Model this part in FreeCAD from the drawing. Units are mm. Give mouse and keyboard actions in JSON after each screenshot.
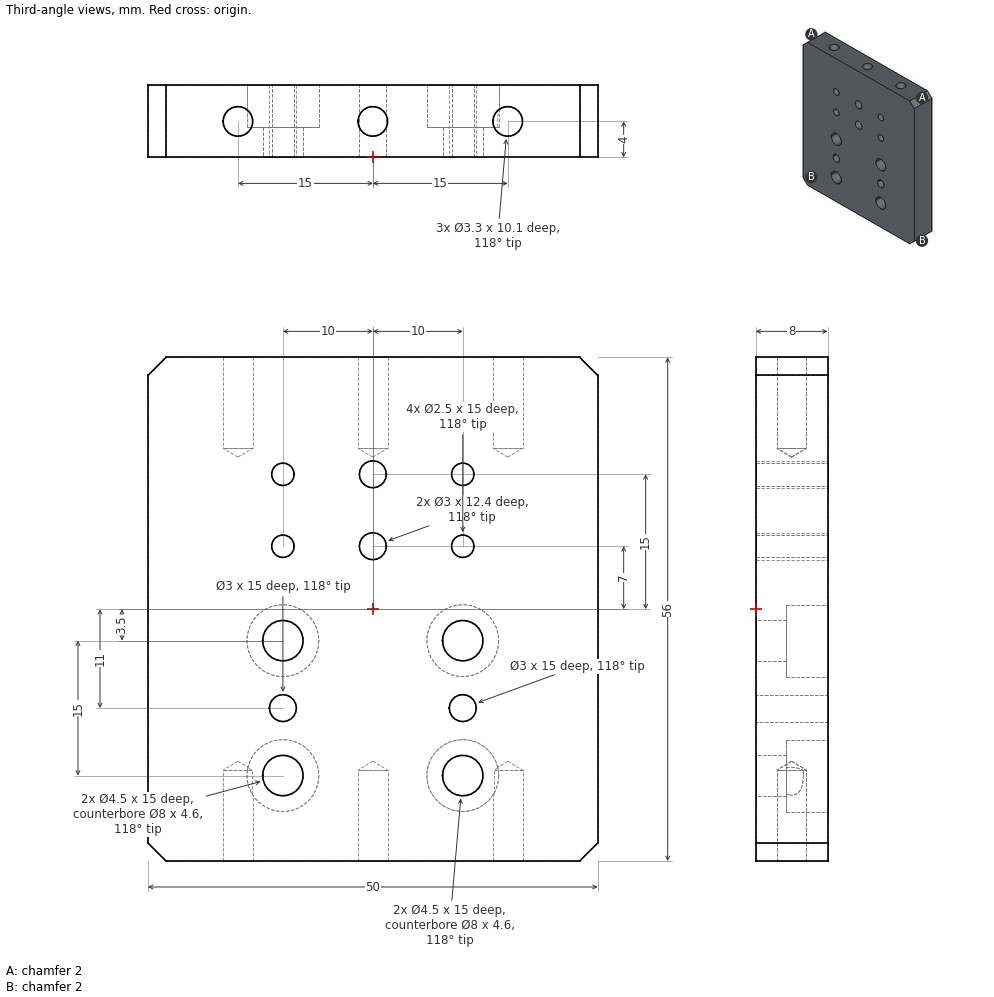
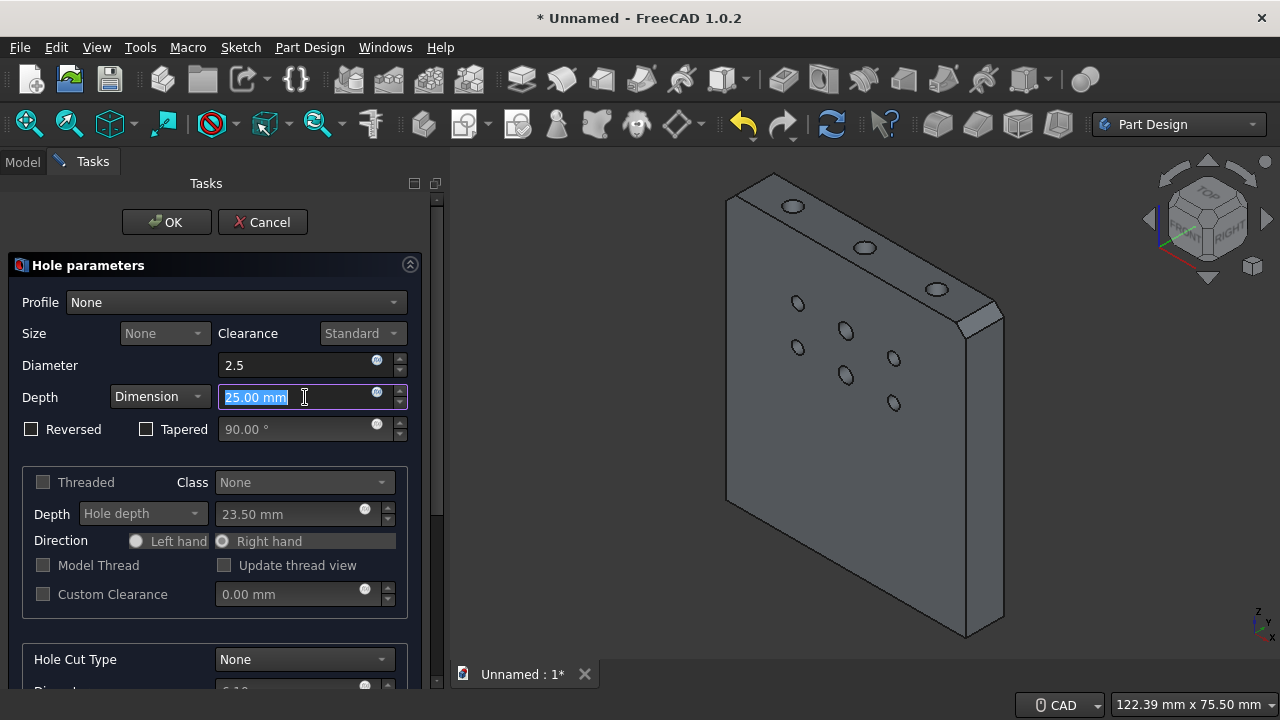
{"action": "type", "text": "15"}
{"action": "key", "text": "Tab"}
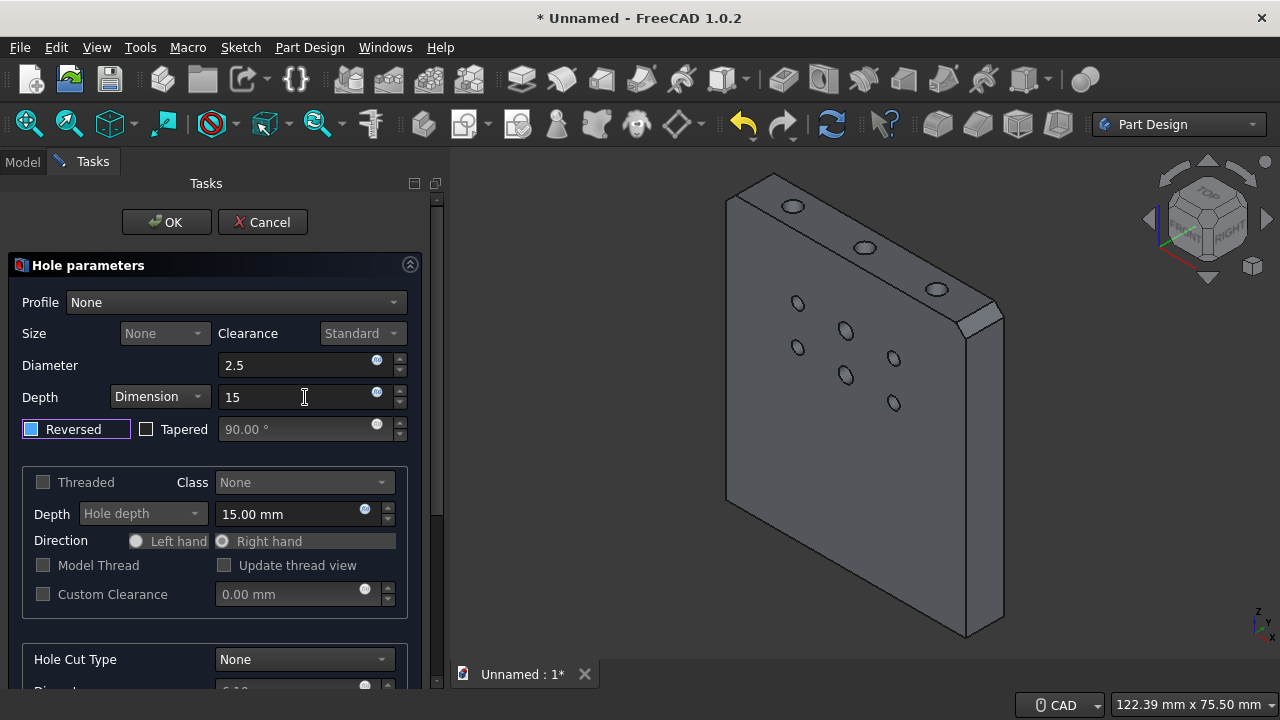
{"action": "left_click", "coordinate": [167, 222]}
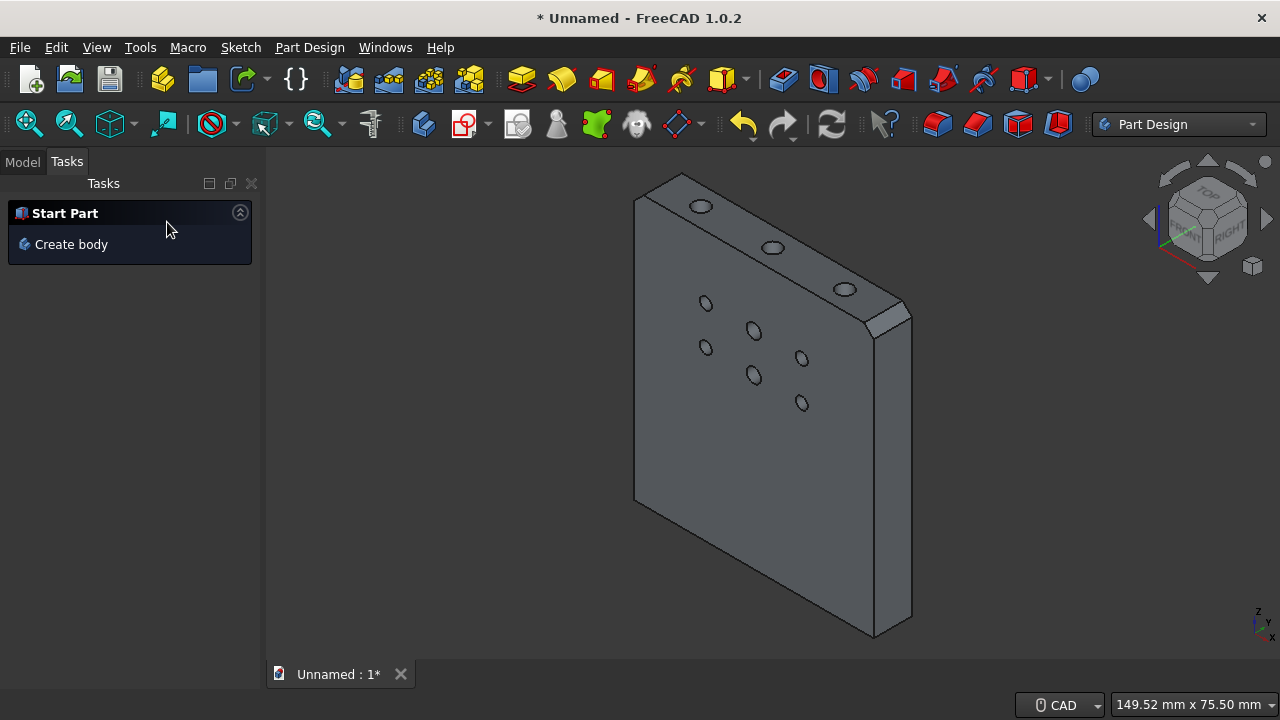
{"action": "key", "text": "4"}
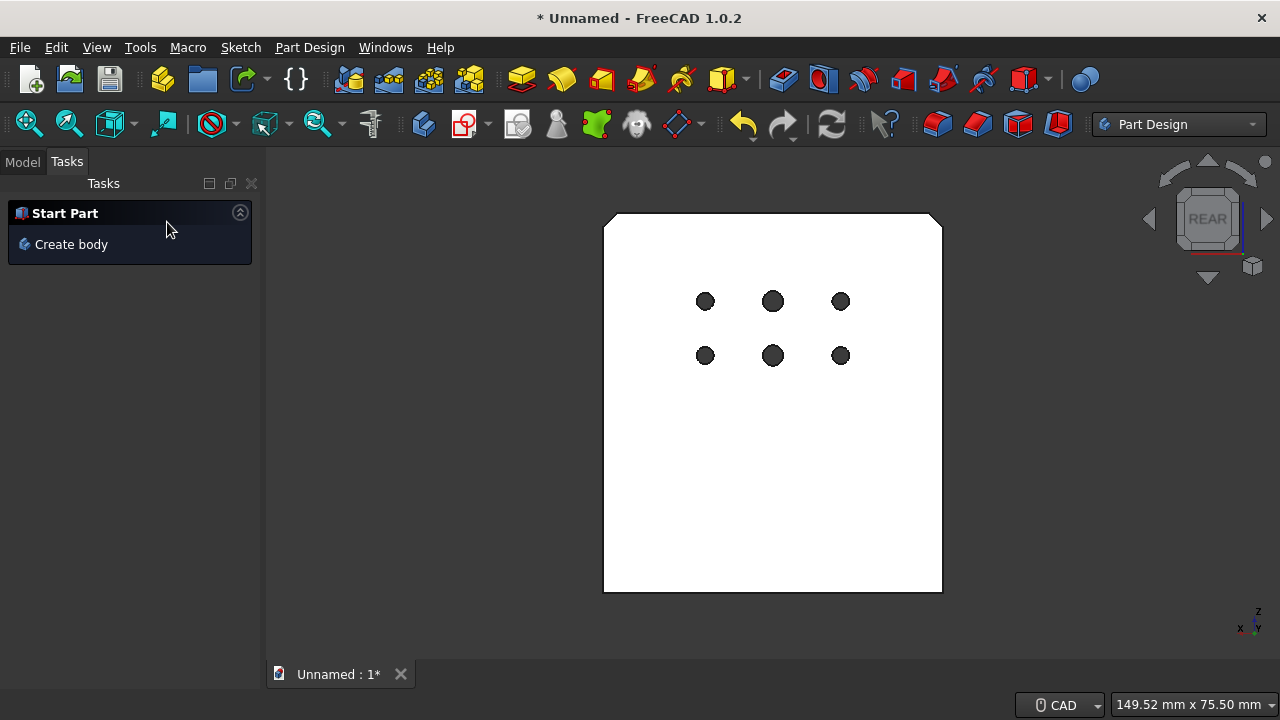
{"action": "left_click", "coordinate": [725, 456]}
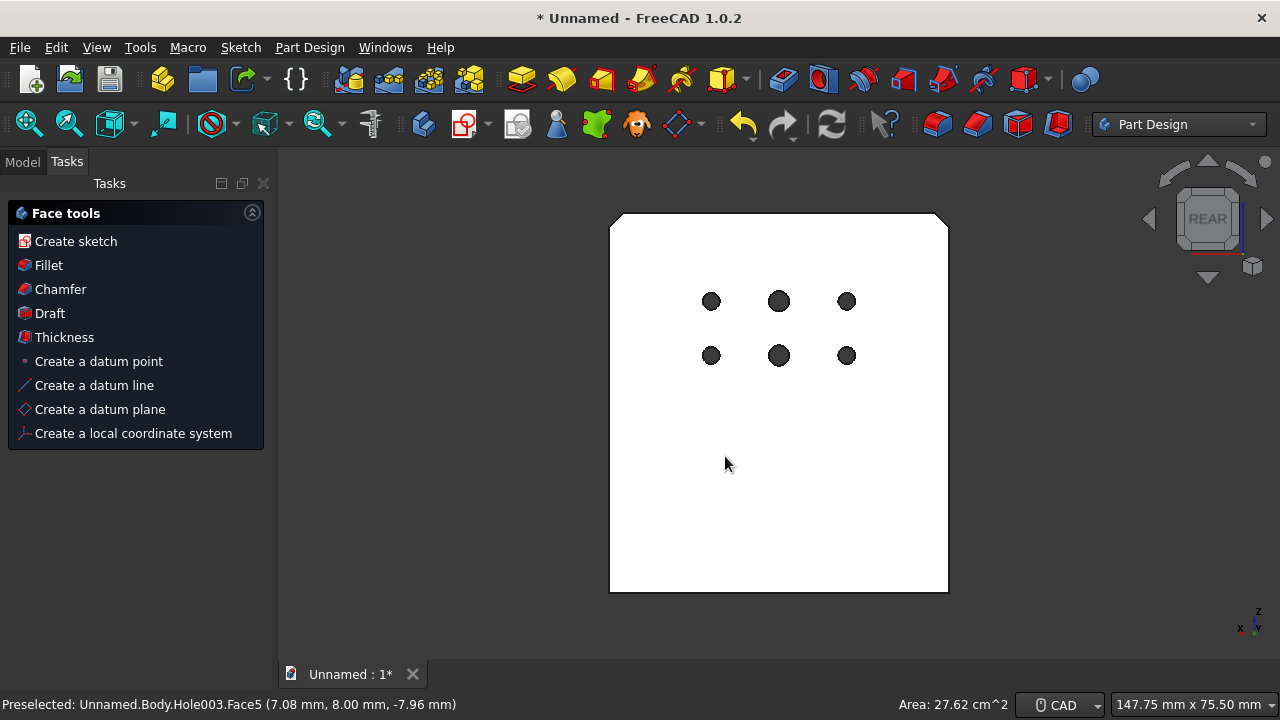
{"action": "left_click", "coordinate": [464, 124]}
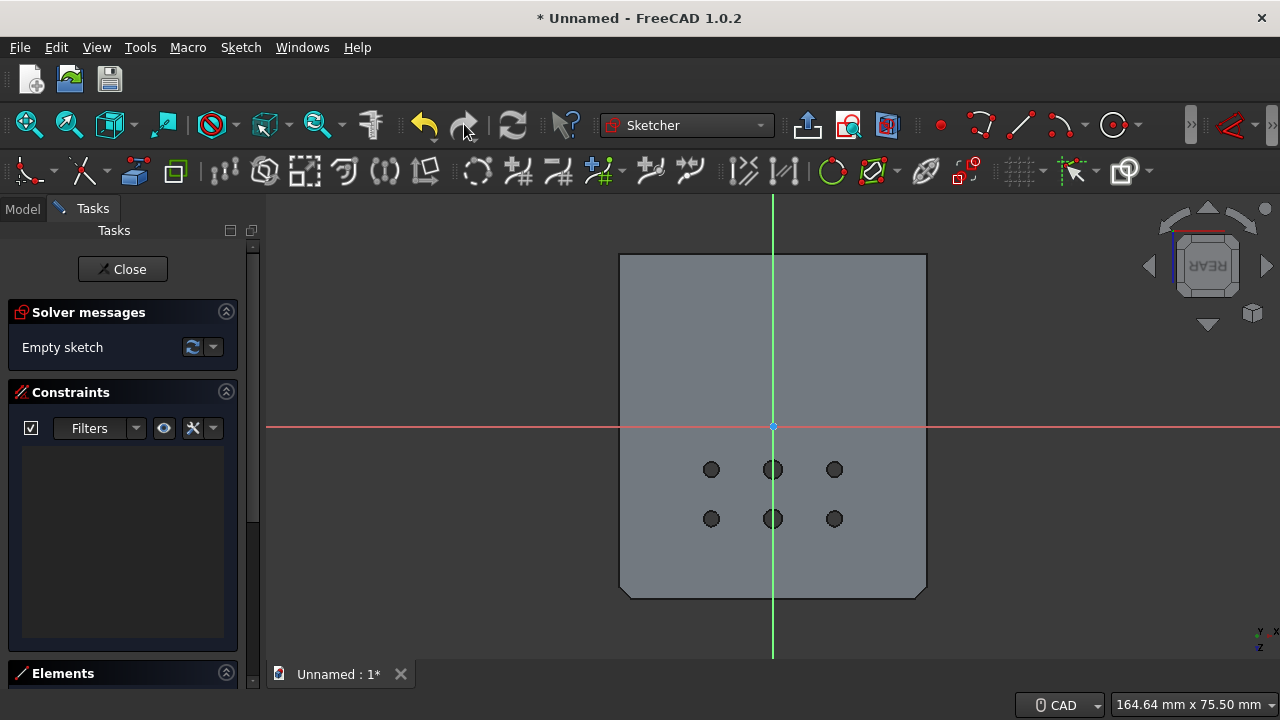
{"action": "scroll", "coordinate": [712, 354], "scroll_direction": "up", "scroll_amount": 14}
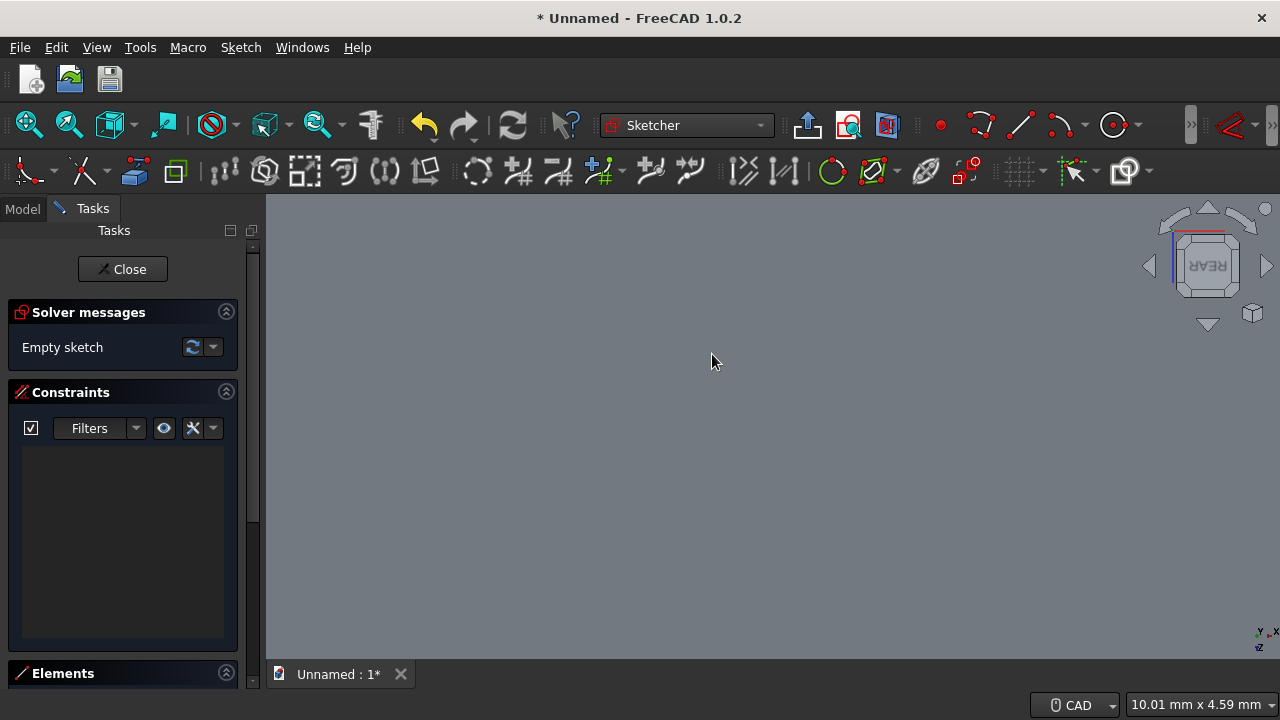
{"action": "key", "text": "g c"}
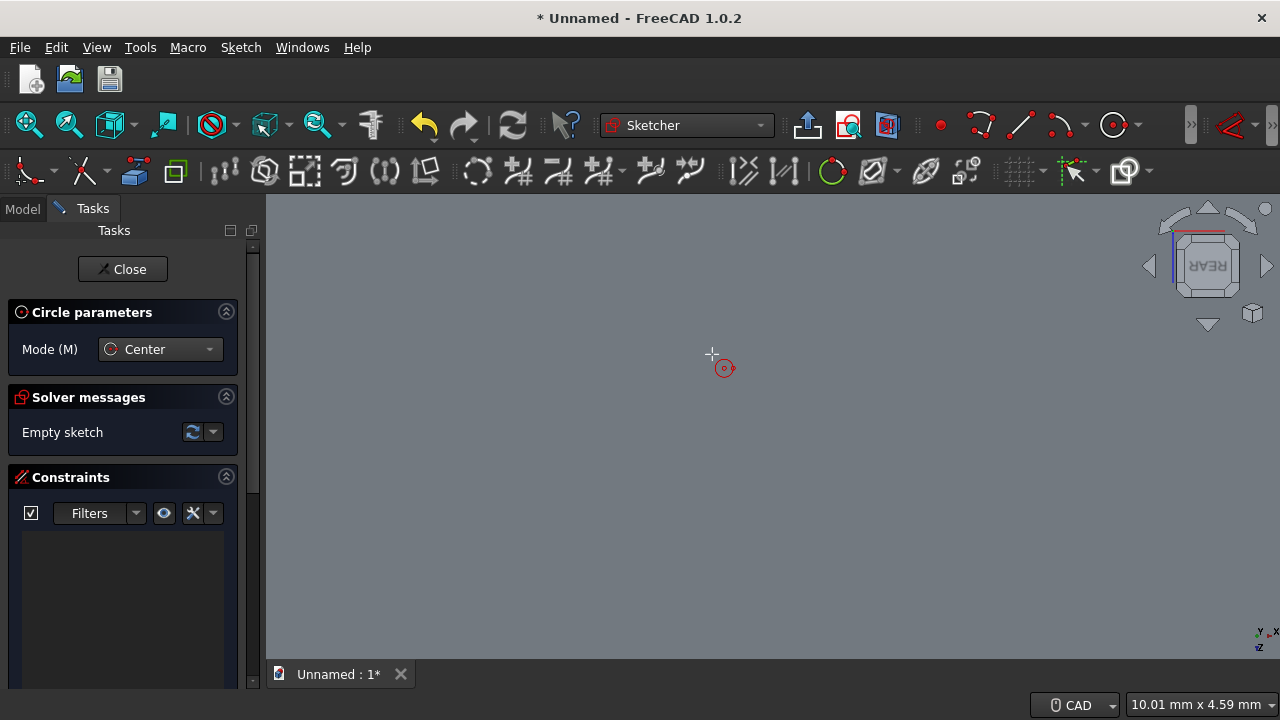
{"action": "left_click", "coordinate": [695, 427]}
{"action": "mouse_move", "coordinate": [803, 319]}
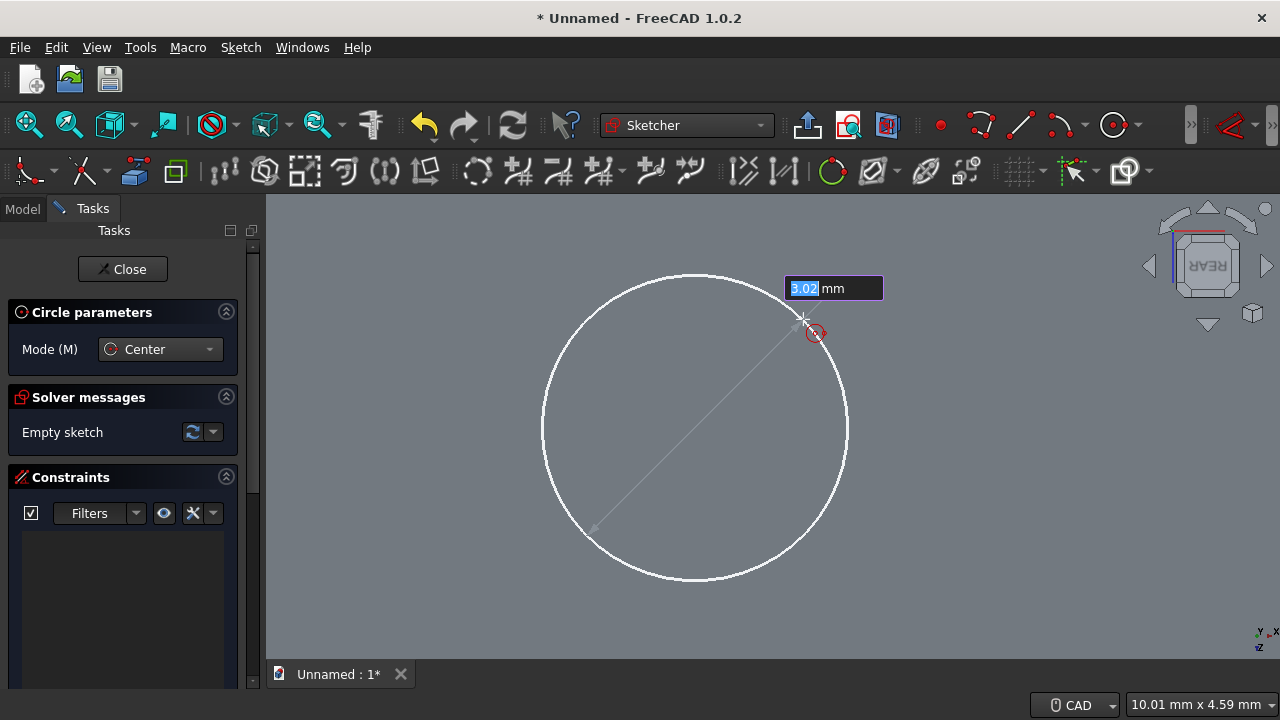
{"action": "type", "text": "3"}
{"action": "key", "text": "Return"}
{"action": "key", "text": "Escape"}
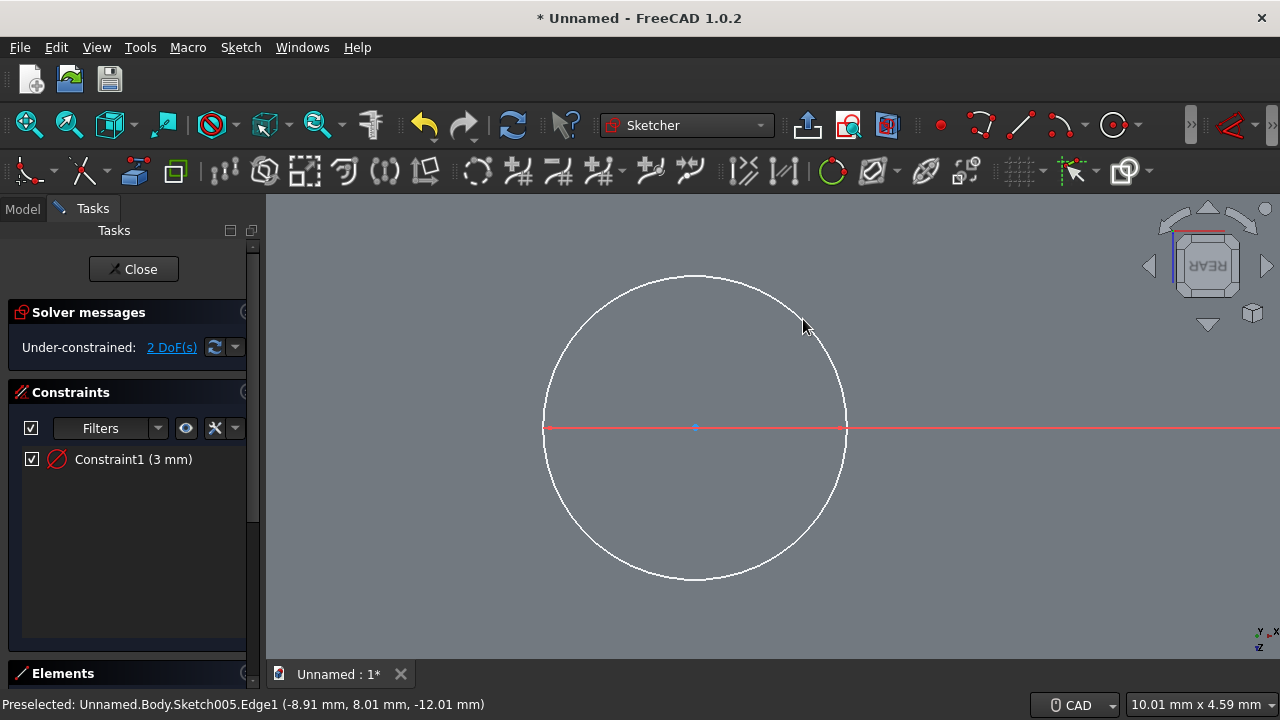
{"action": "left_click", "coordinate": [1230, 126]}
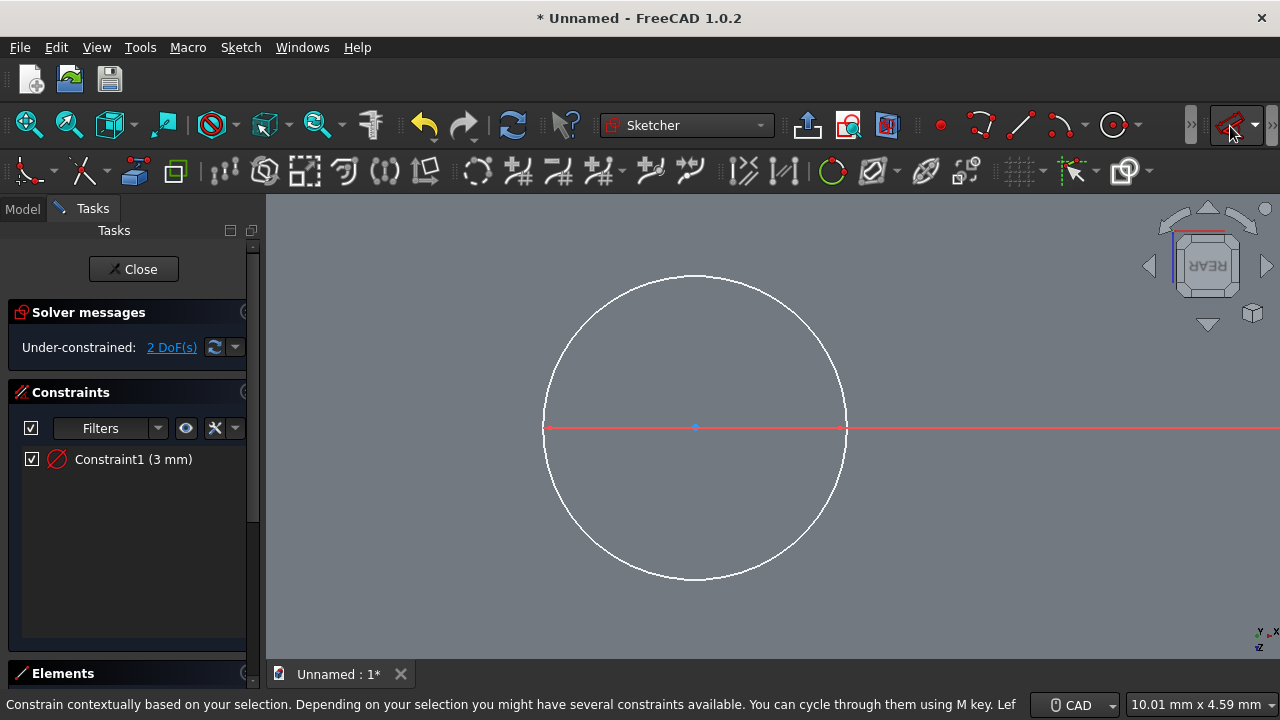
{"action": "left_click", "coordinate": [695, 428]}
{"action": "left_click", "coordinate": [905, 394]}